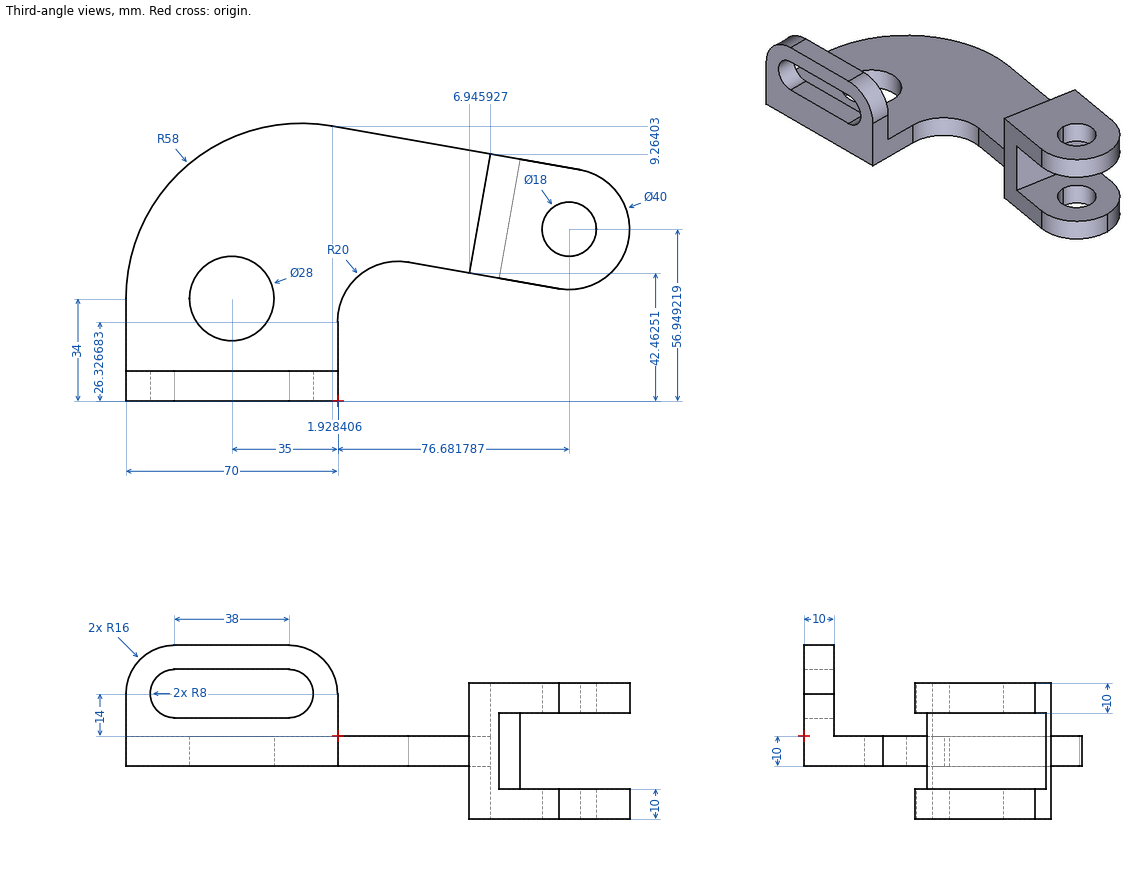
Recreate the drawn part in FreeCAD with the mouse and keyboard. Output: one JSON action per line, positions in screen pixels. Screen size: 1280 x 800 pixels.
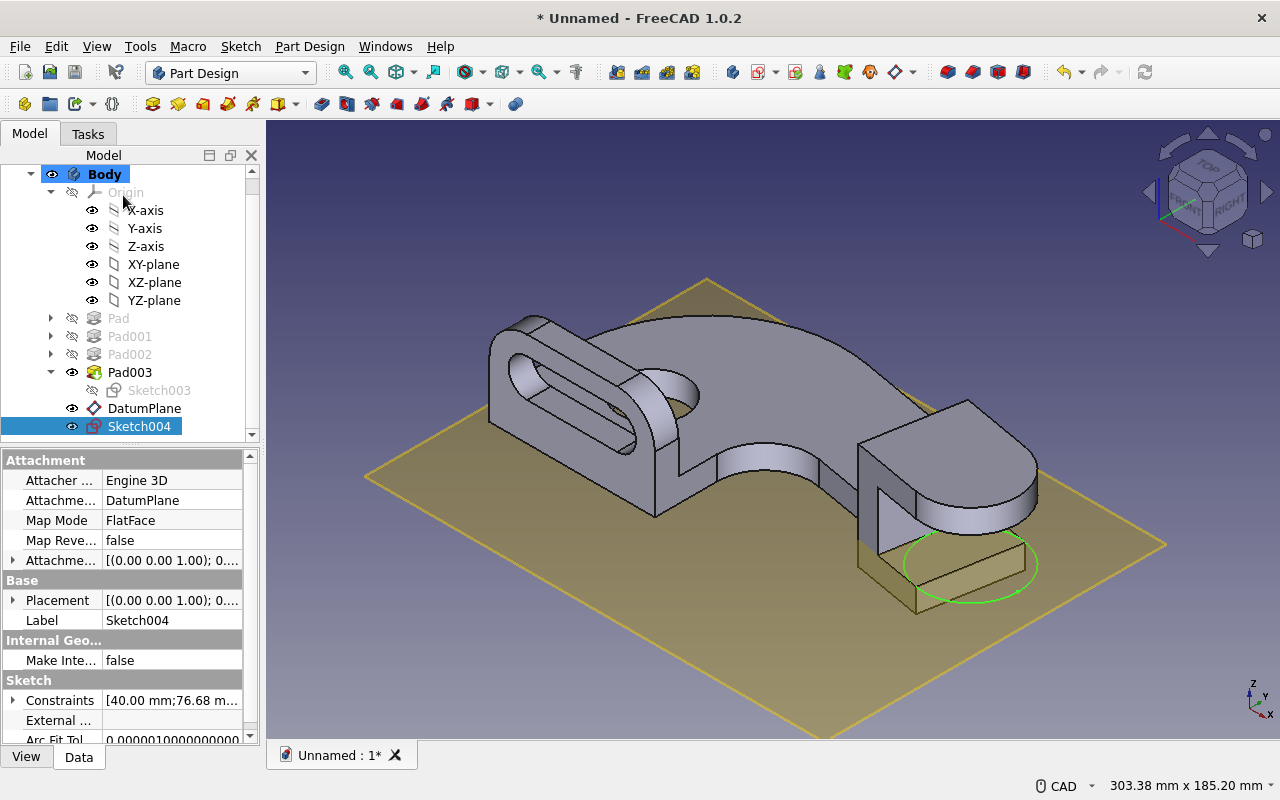
{"action": "left_click", "coordinate": [153, 104]}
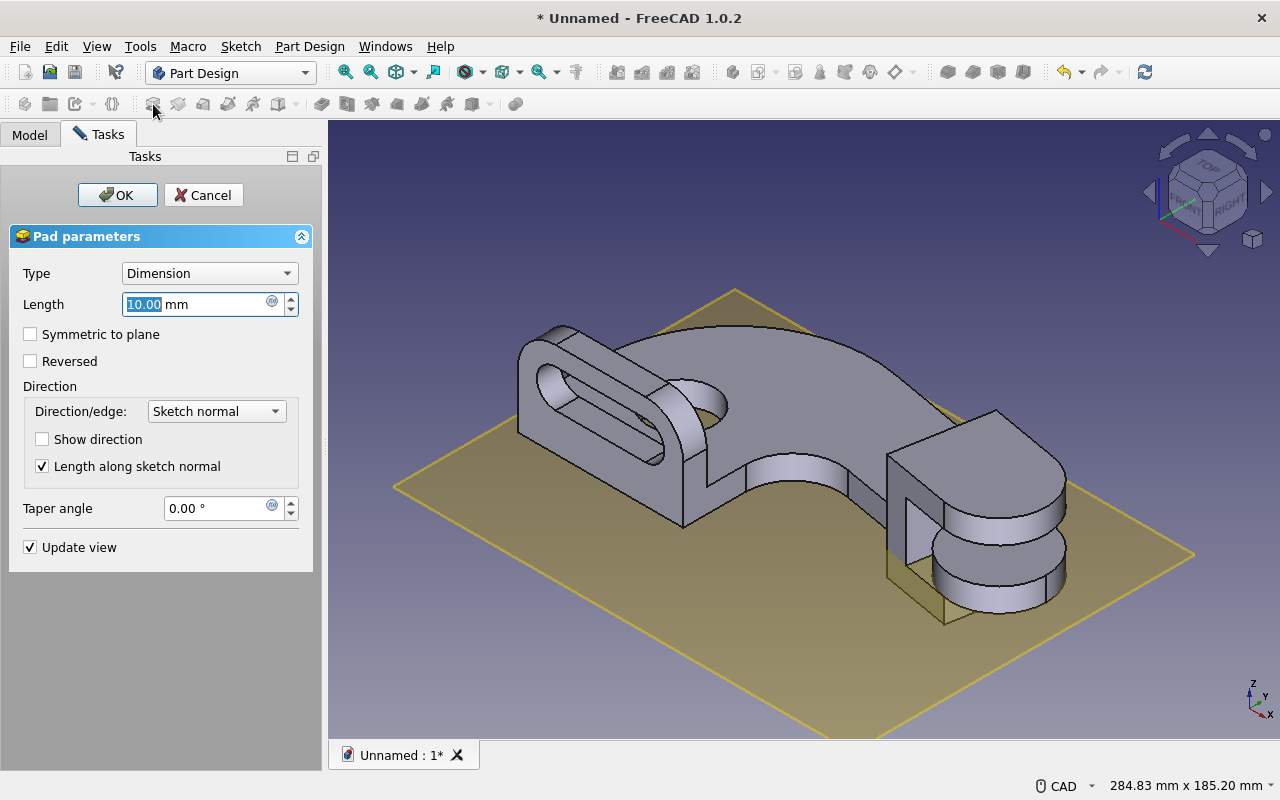
{"action": "type", "text": "10"}
{"action": "key", "text": "Tab"}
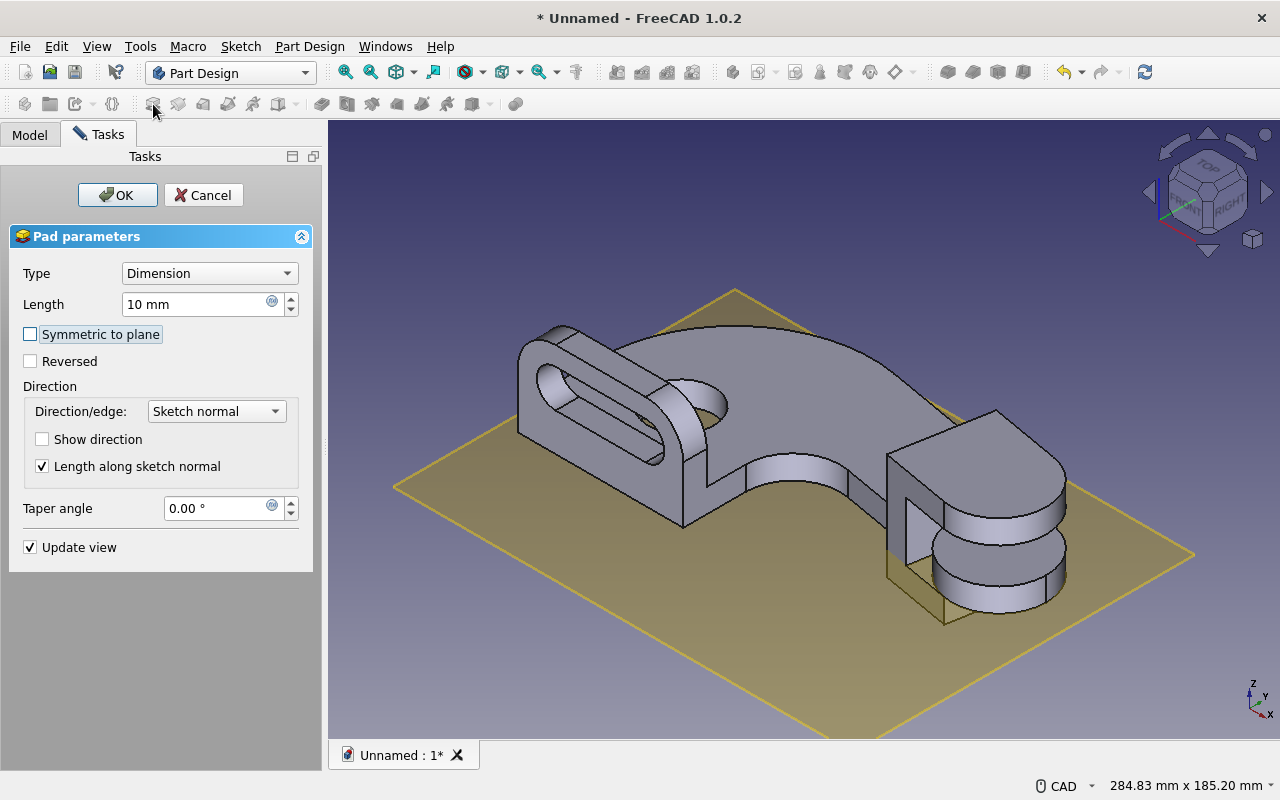
{"action": "left_click", "coordinate": [31, 361]}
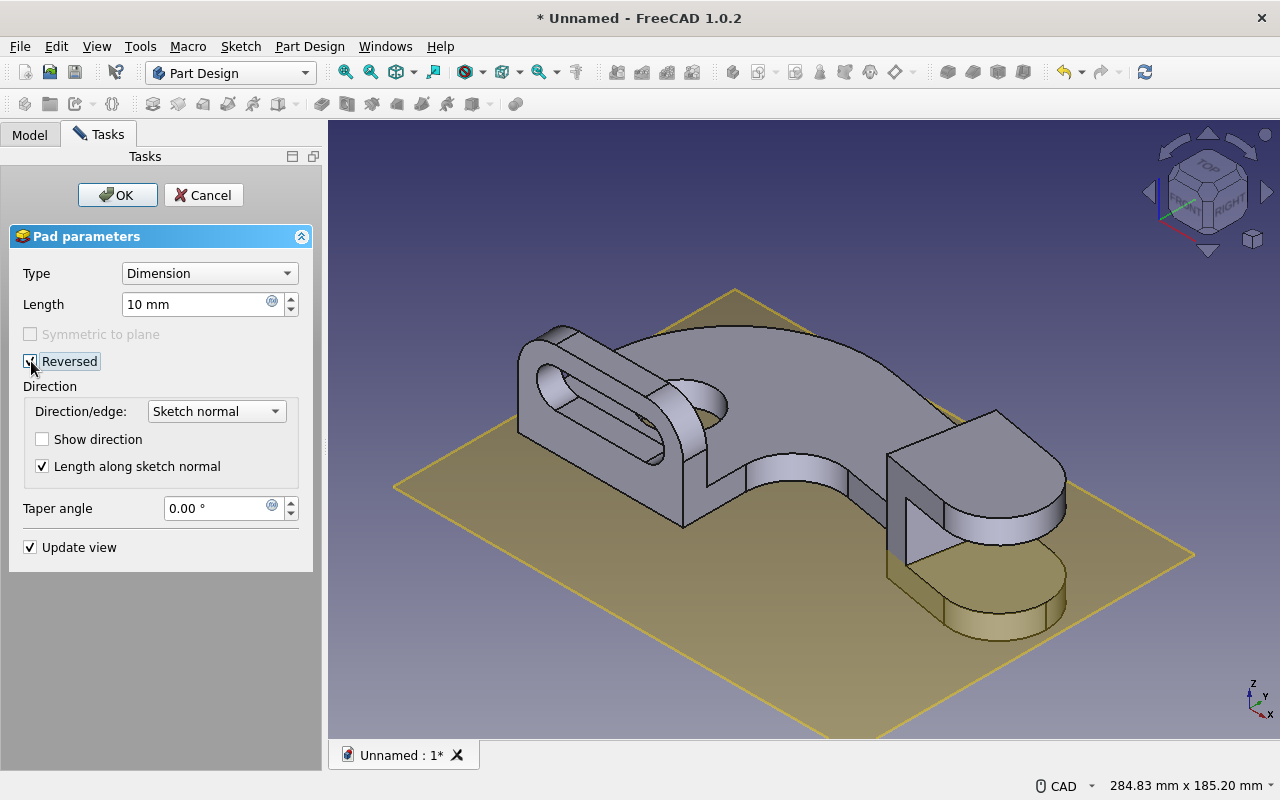
{"action": "left_click", "coordinate": [118, 195]}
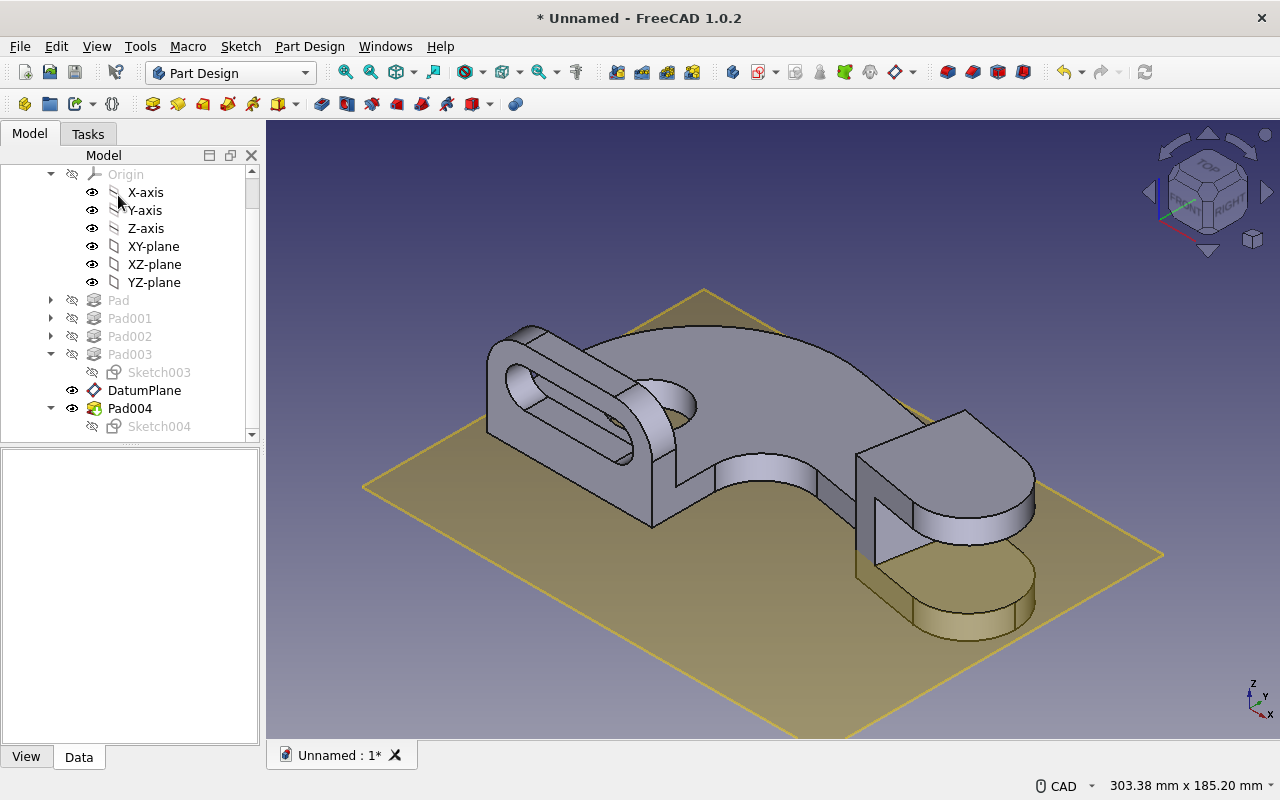
{"action": "left_click", "coordinate": [117, 390]}
{"action": "key", "text": "space"}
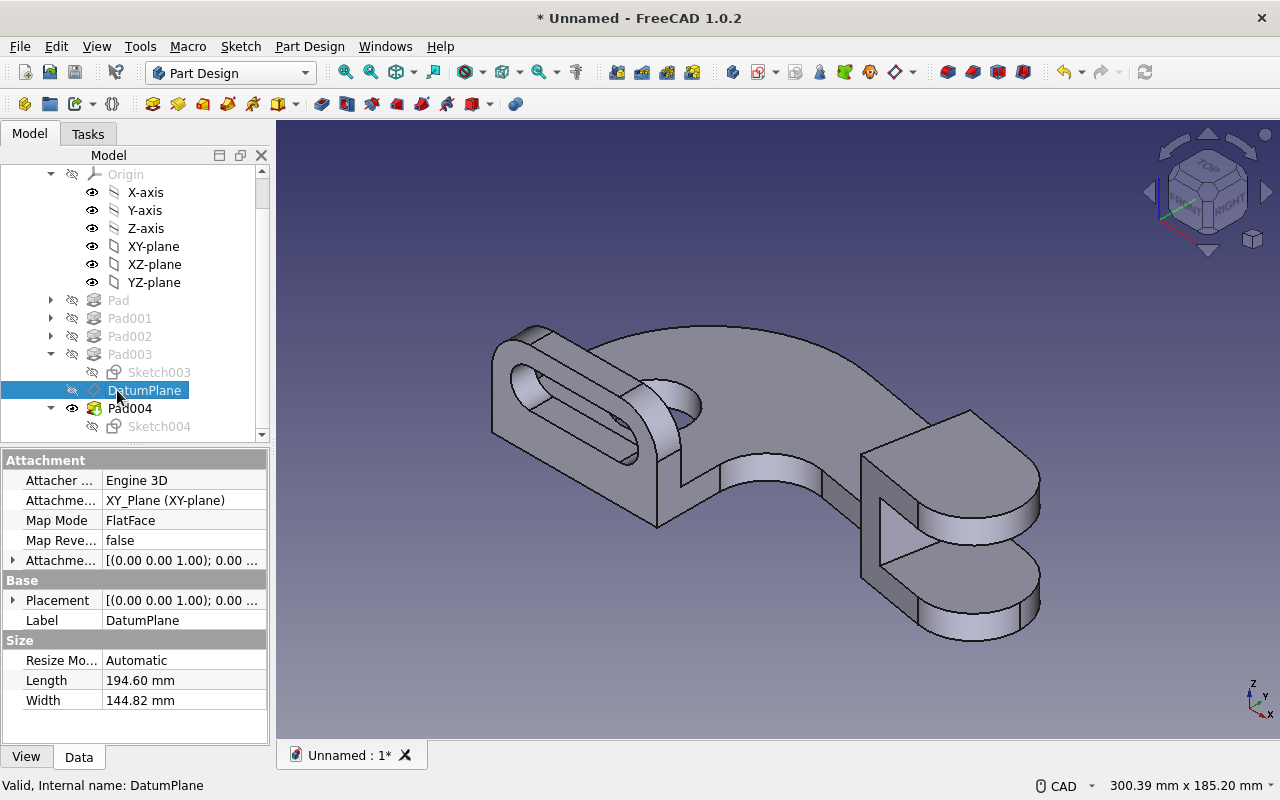
{"action": "left_click", "coordinate": [964, 466]}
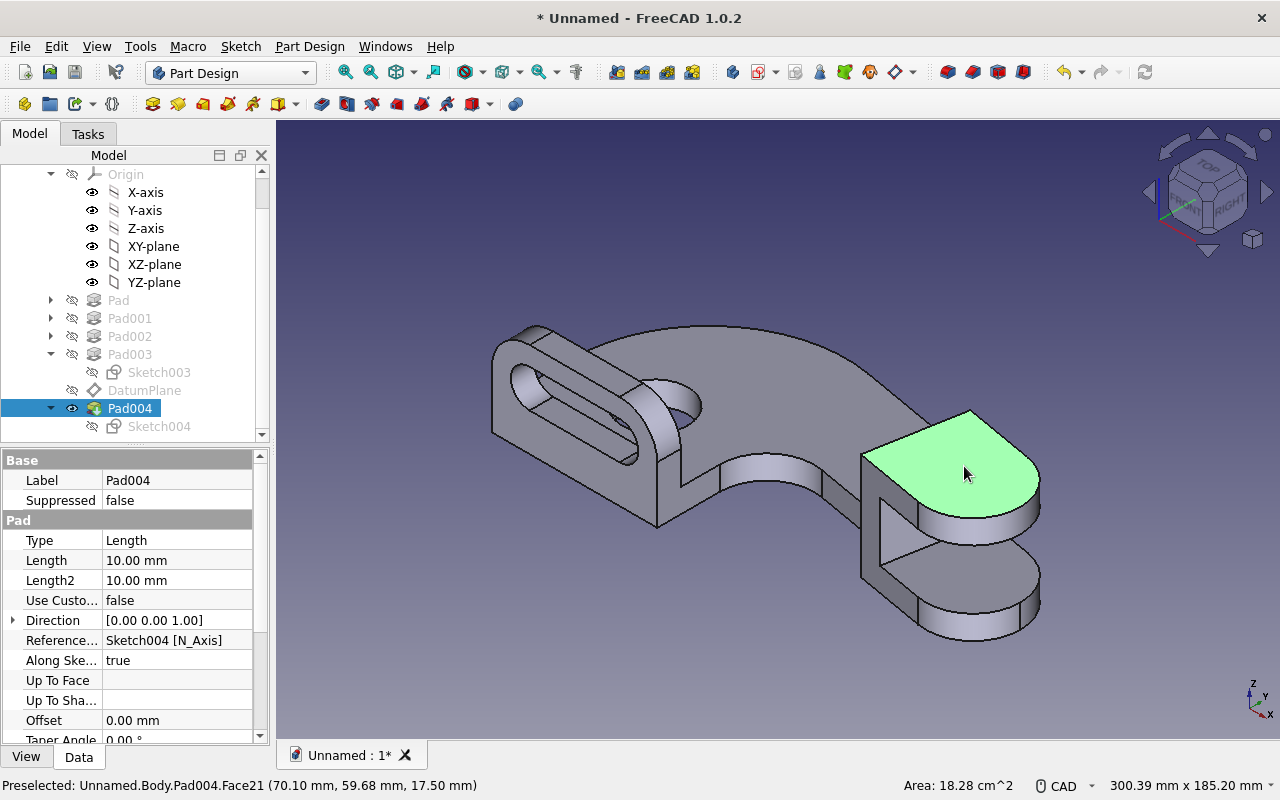
{"action": "left_click", "coordinate": [758, 72]}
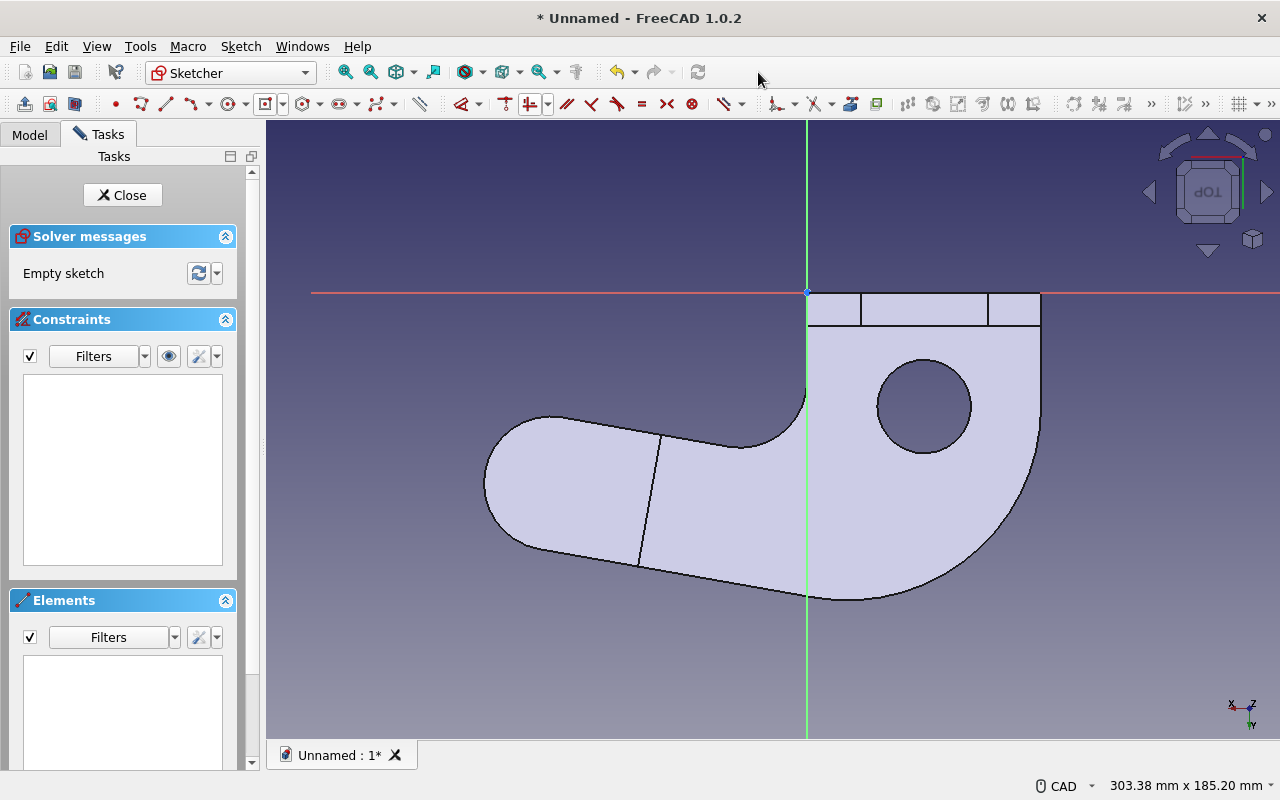
{"action": "key", "text": "q s"}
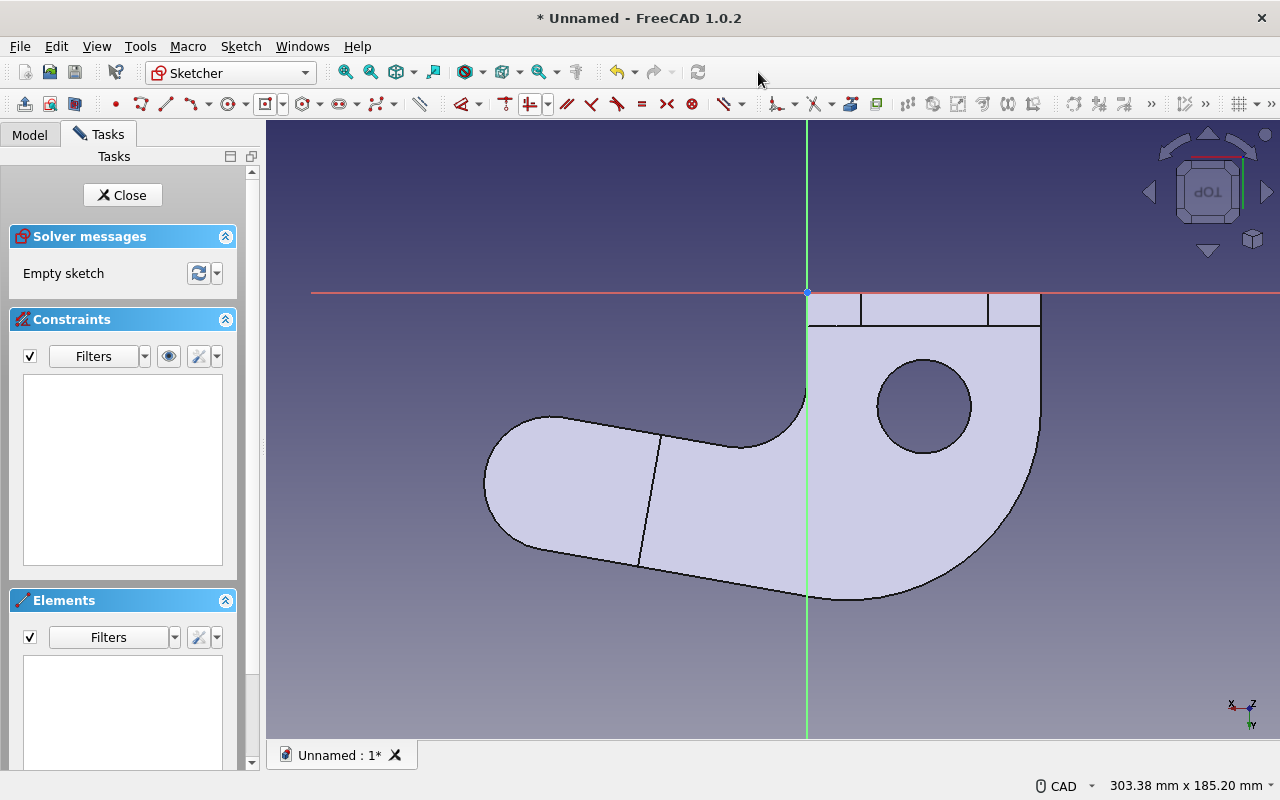
{"action": "scroll", "coordinate": [520, 494], "scroll_direction": "up", "scroll_amount": 9}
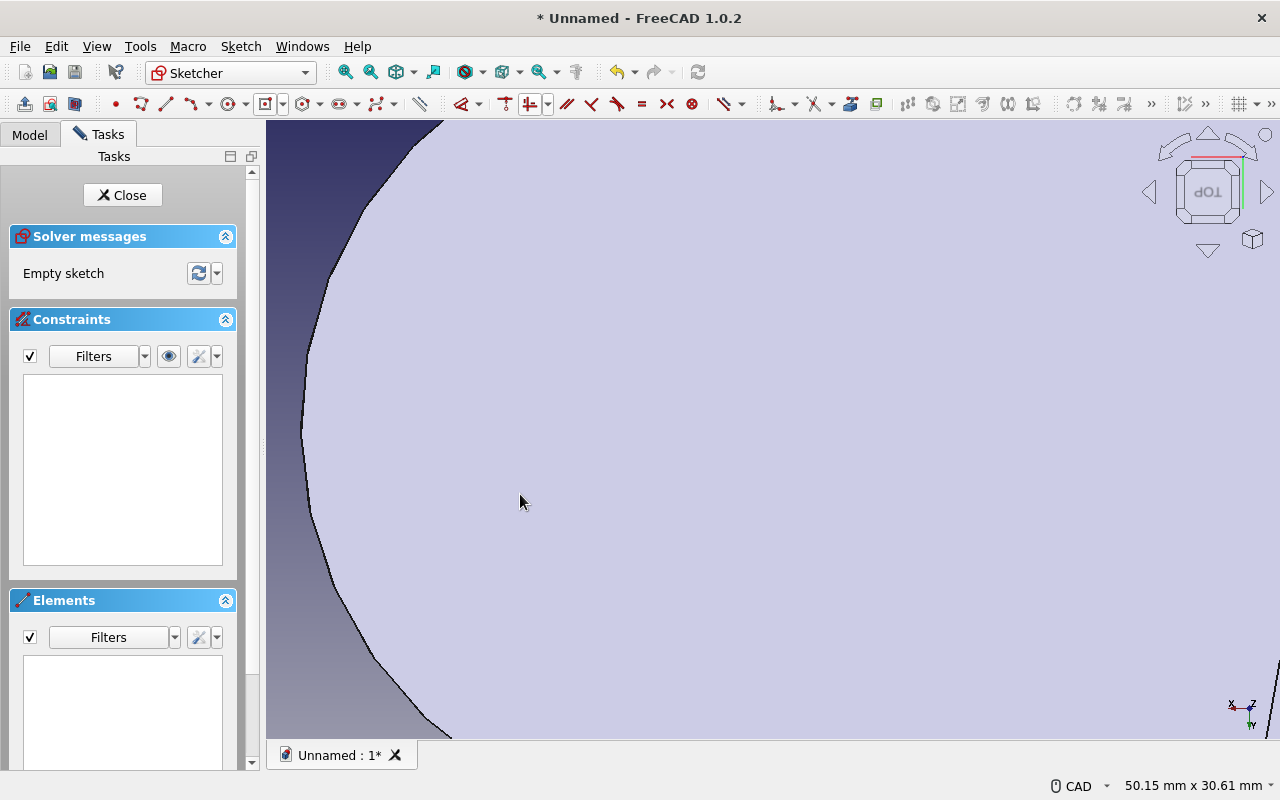
{"action": "left_click", "coordinate": [228, 104]}